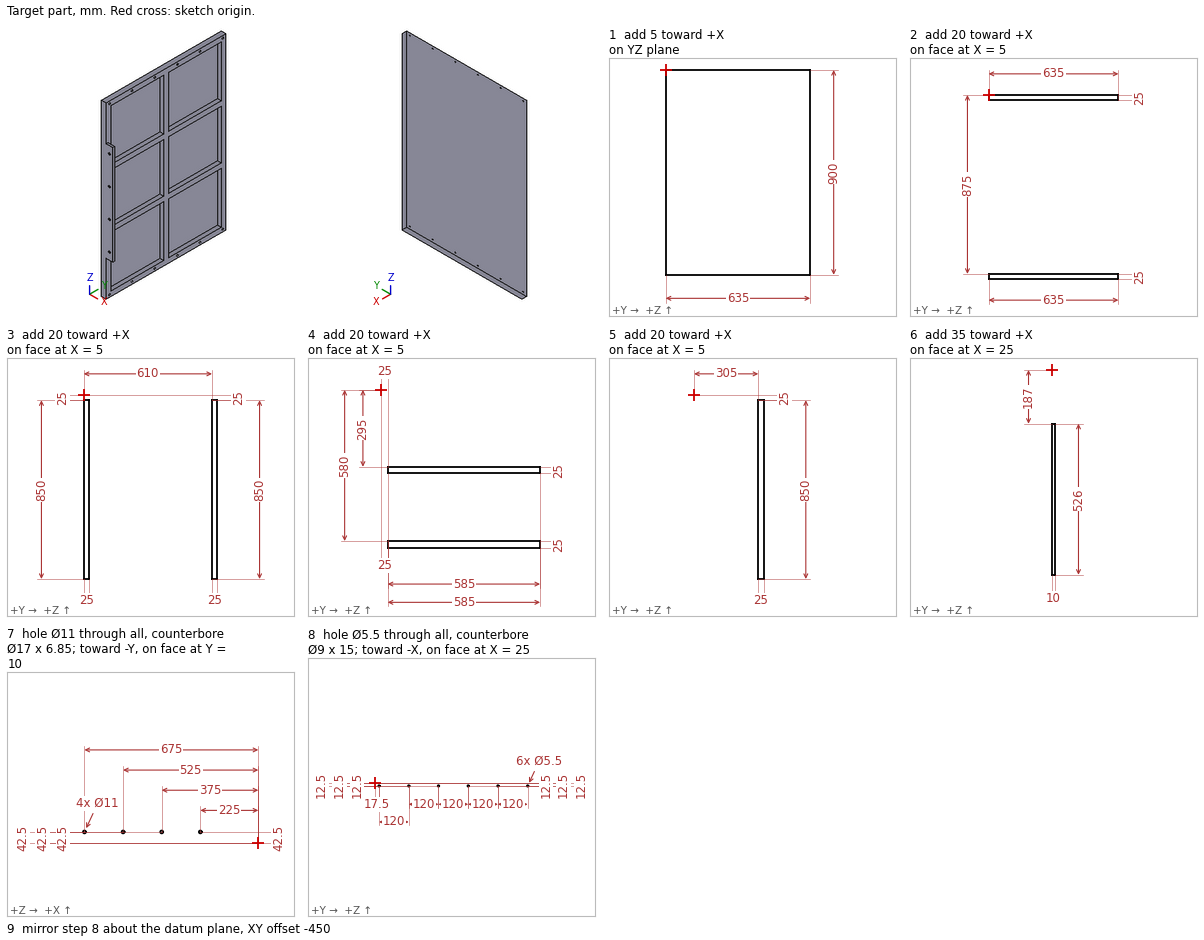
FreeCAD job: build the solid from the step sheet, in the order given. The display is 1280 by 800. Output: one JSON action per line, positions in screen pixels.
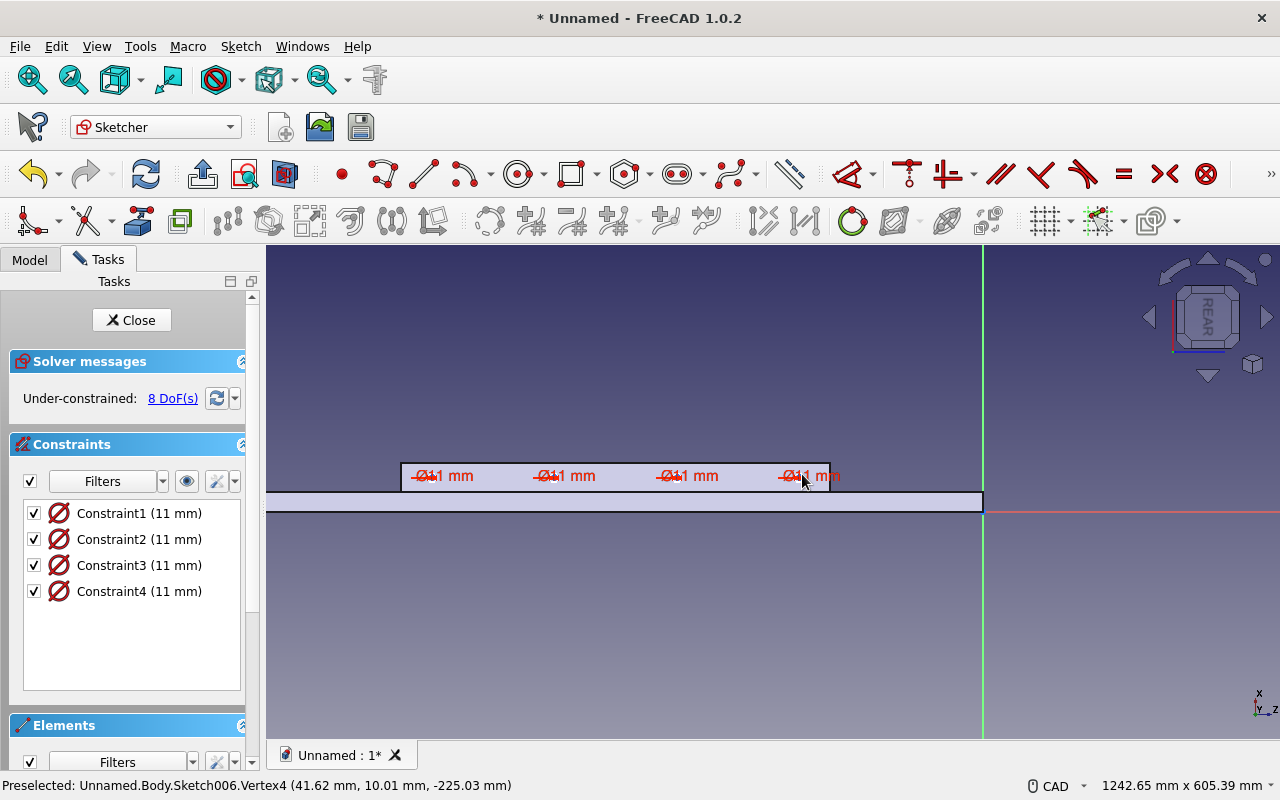
{"action": "key", "text": "d"}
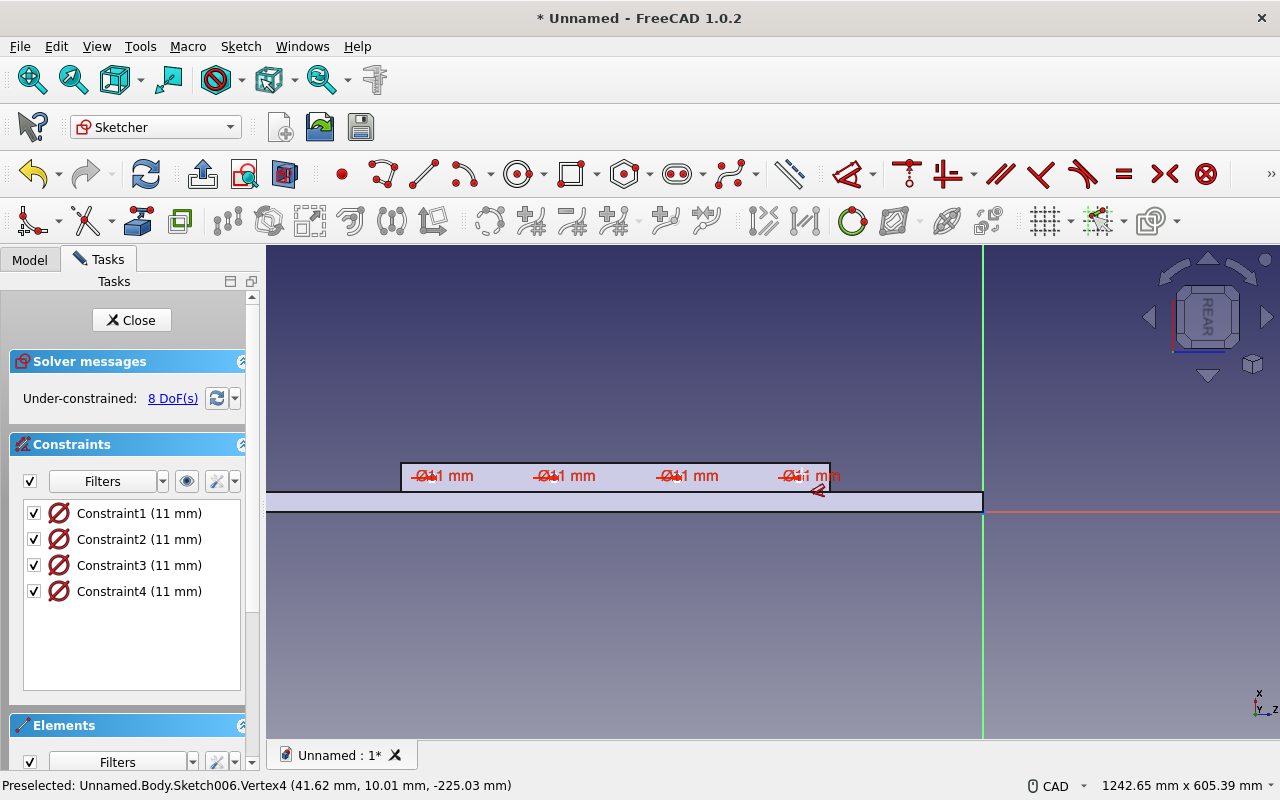
{"action": "left_click", "coordinate": [432, 478]}
{"action": "left_click", "coordinate": [707, 546]}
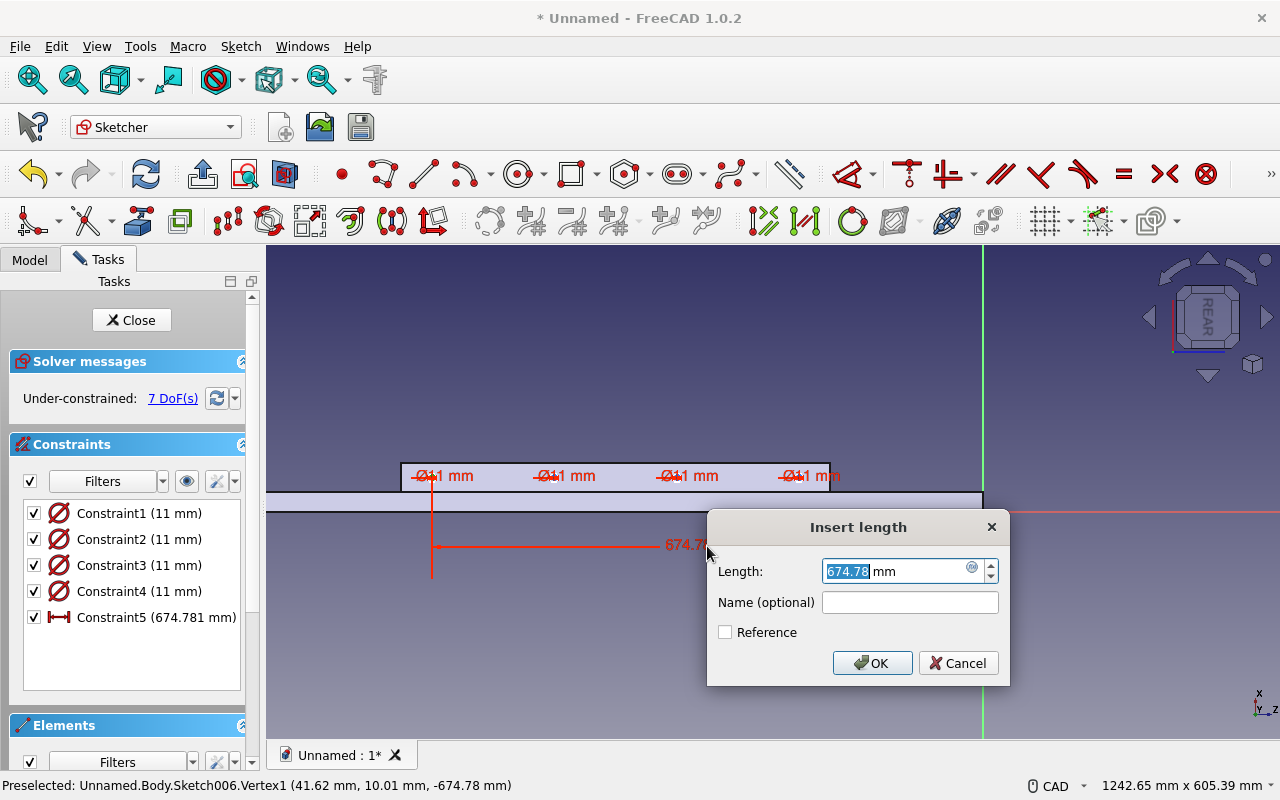
{"action": "type", "text": "675"}
{"action": "key", "text": "Return"}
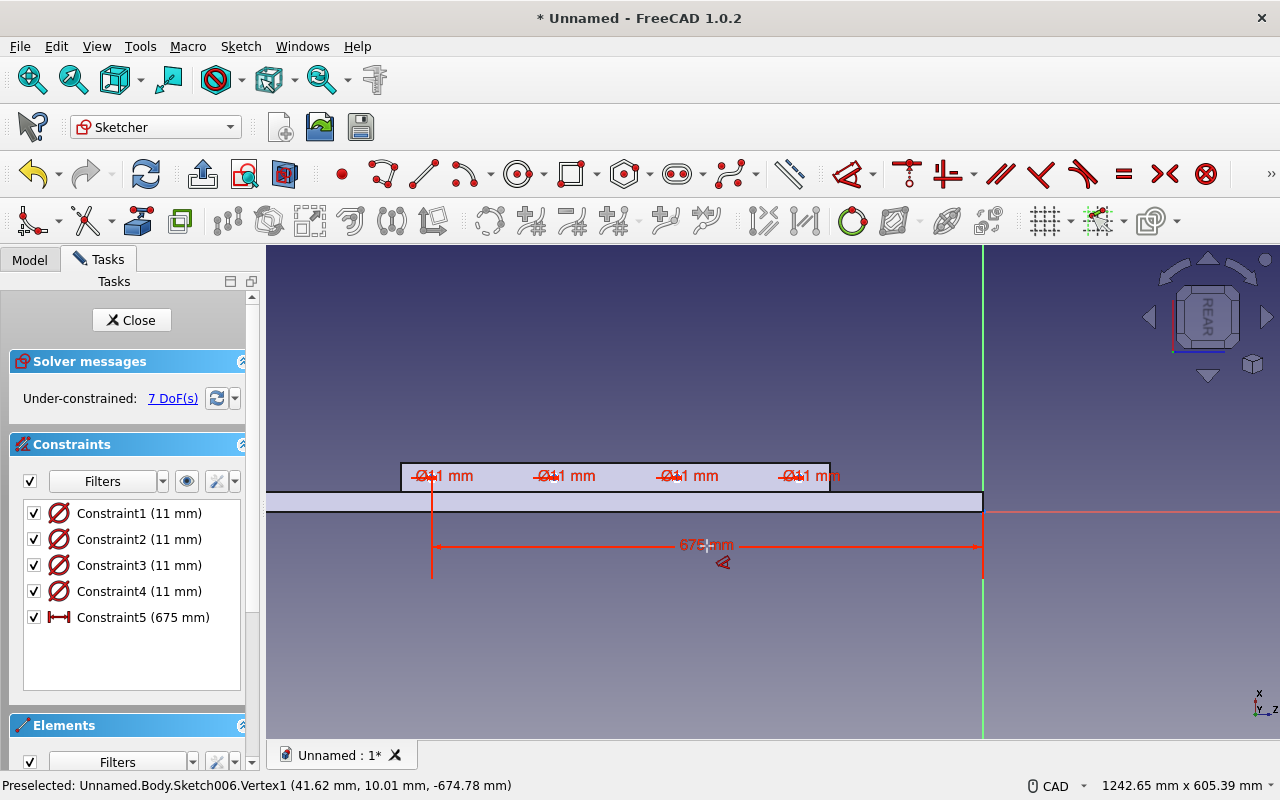
{"action": "left_click", "coordinate": [554, 478]}
{"action": "left_click", "coordinate": [867, 546]}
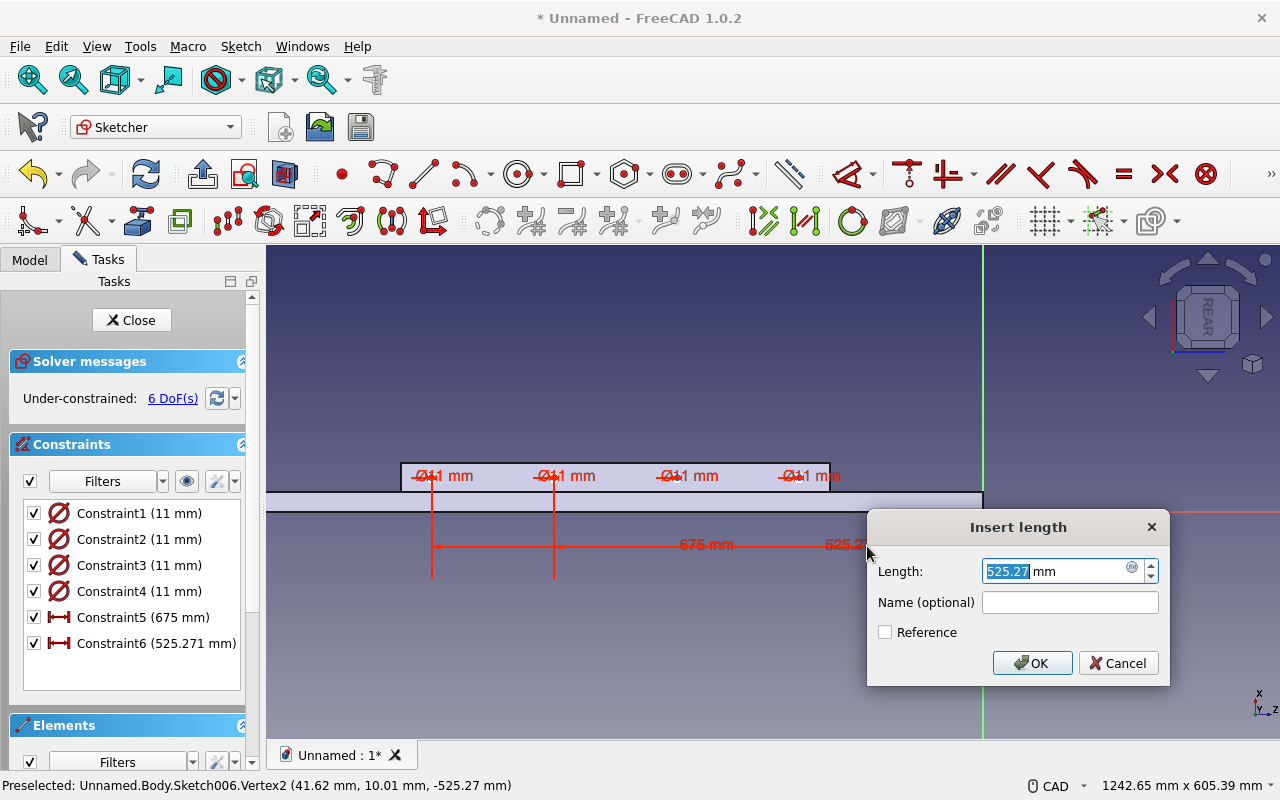
{"action": "type", "text": "525"}
{"action": "key", "text": "Return"}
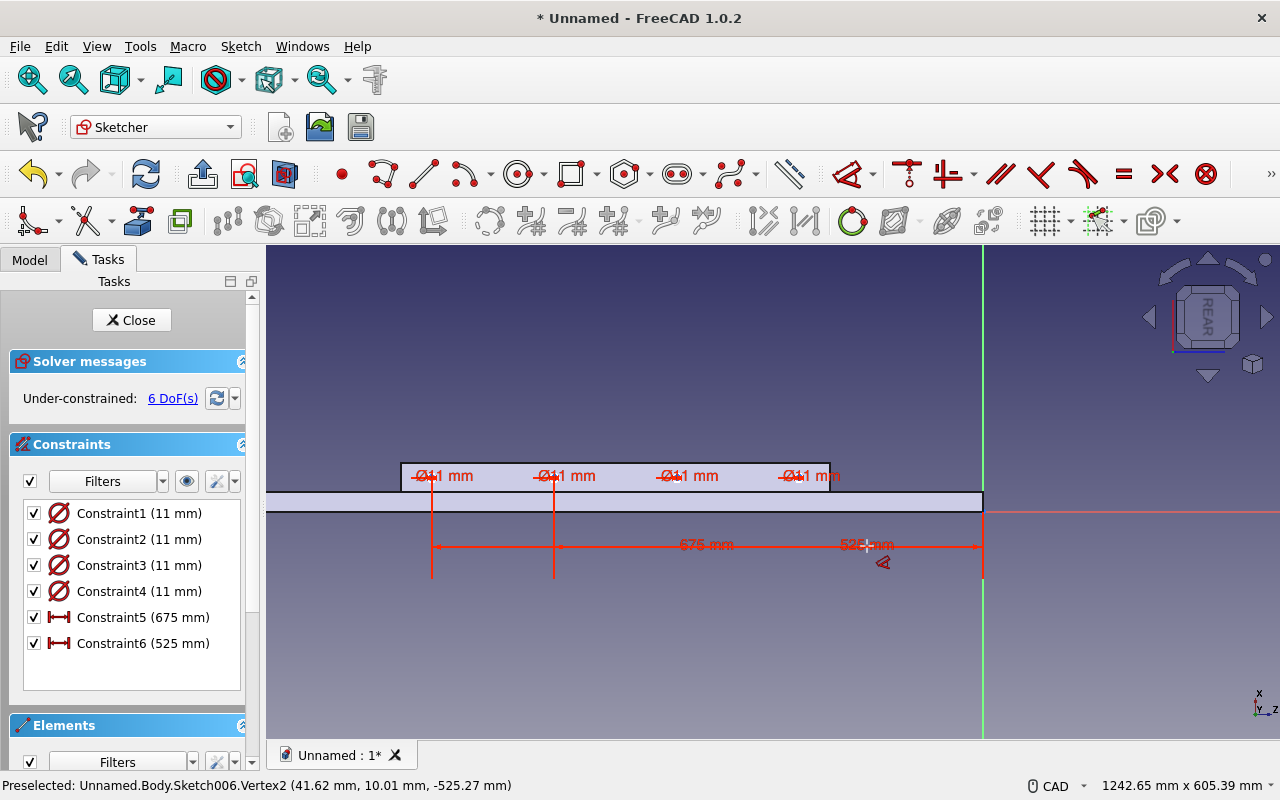
{"action": "left_click", "coordinate": [677, 478]}
{"action": "left_click", "coordinate": [830, 444]}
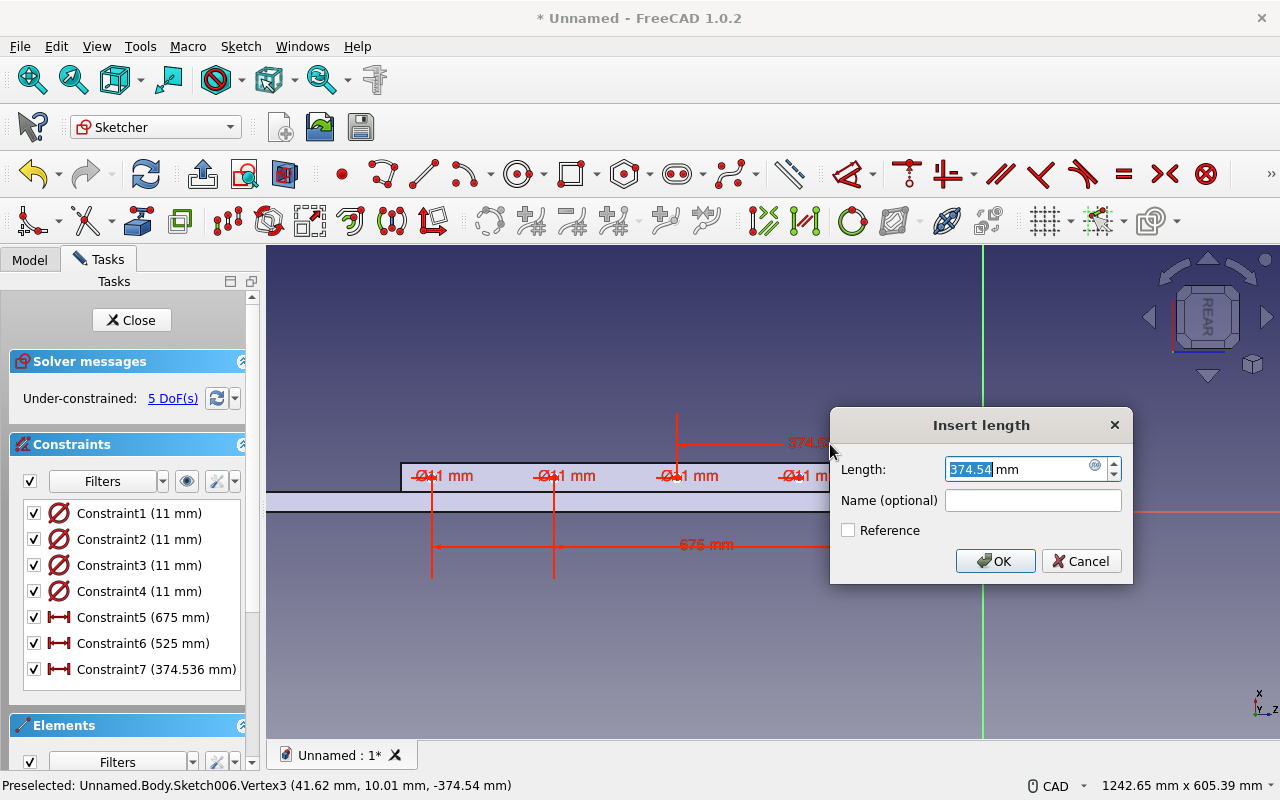
{"action": "type", "text": "375"}
{"action": "key", "text": "Return"}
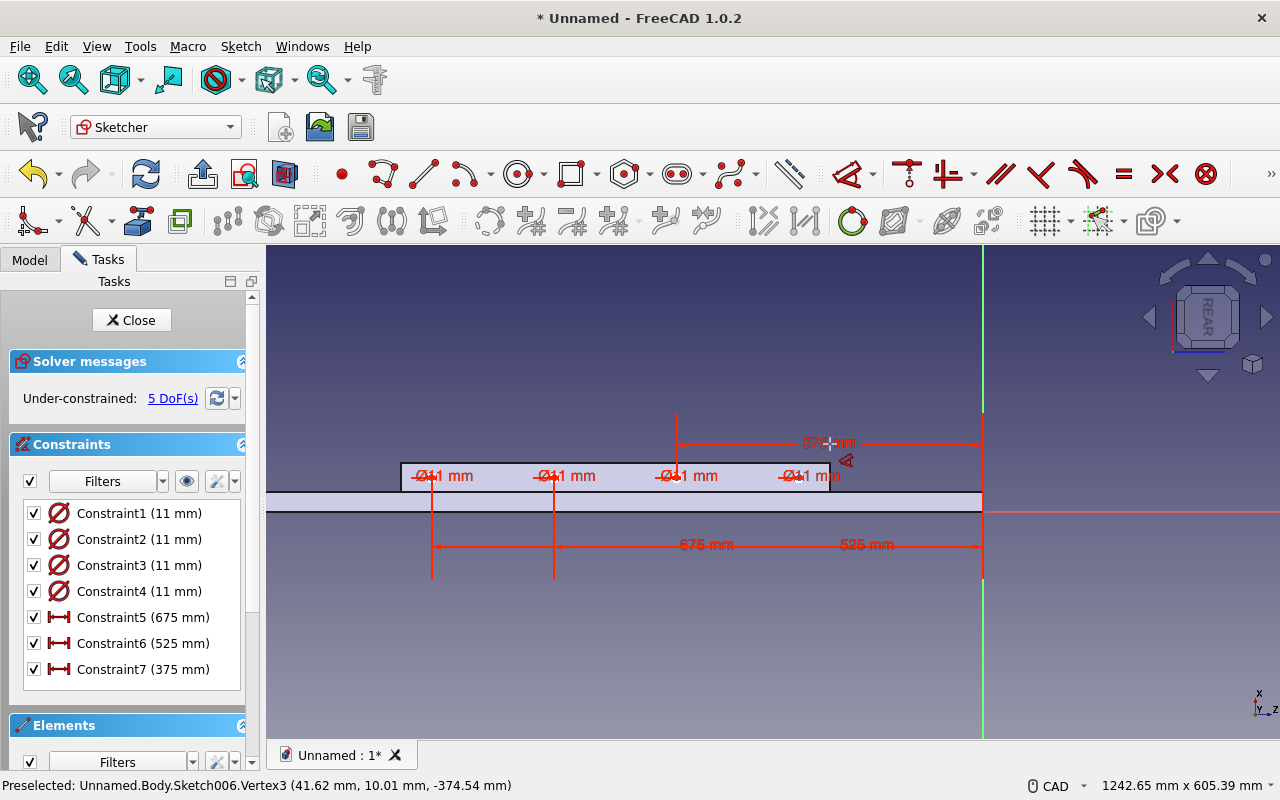
{"action": "left_click", "coordinate": [799, 478]}
{"action": "left_click", "coordinate": [955, 546]}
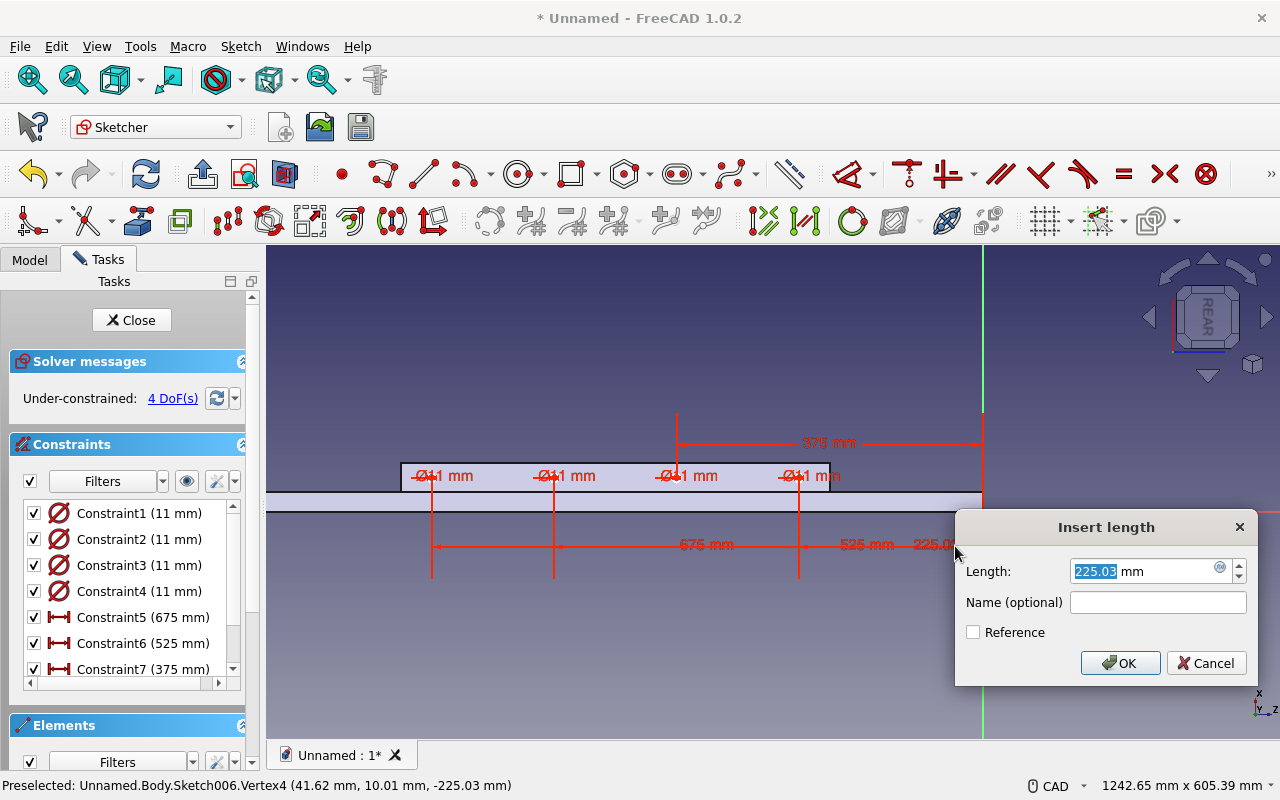
{"action": "type", "text": "225"}
{"action": "key", "text": "Return"}